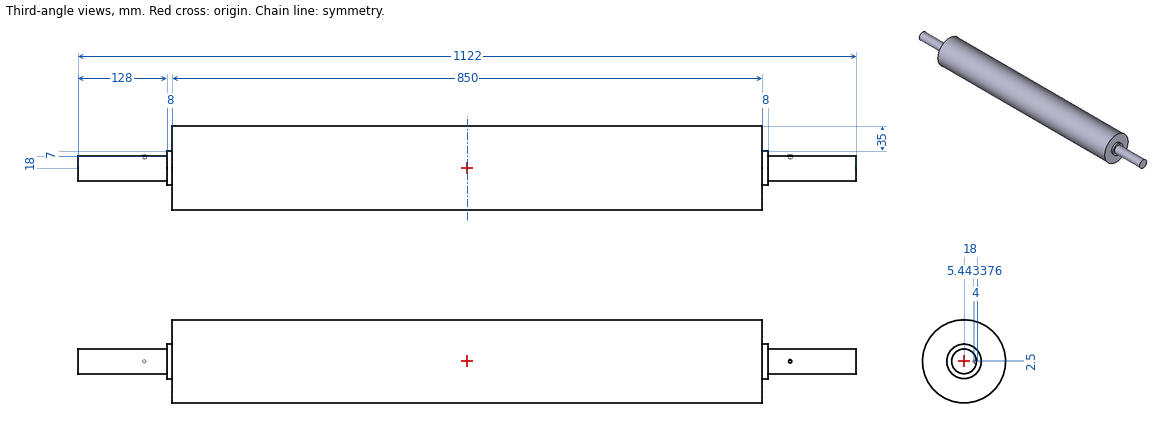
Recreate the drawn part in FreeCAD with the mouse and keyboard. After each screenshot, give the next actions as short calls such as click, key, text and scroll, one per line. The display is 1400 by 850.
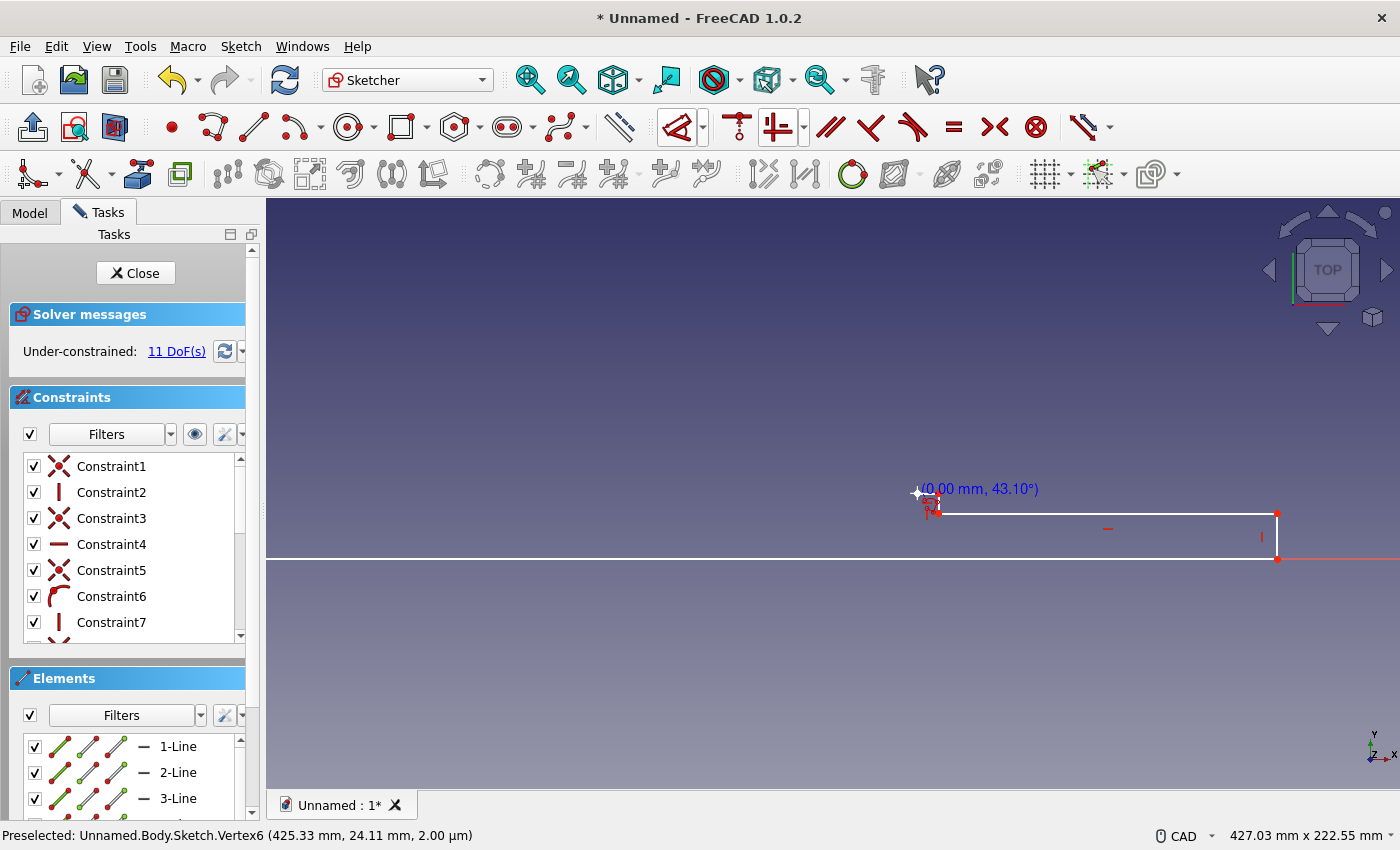
scroll(1011, 497, down, 8)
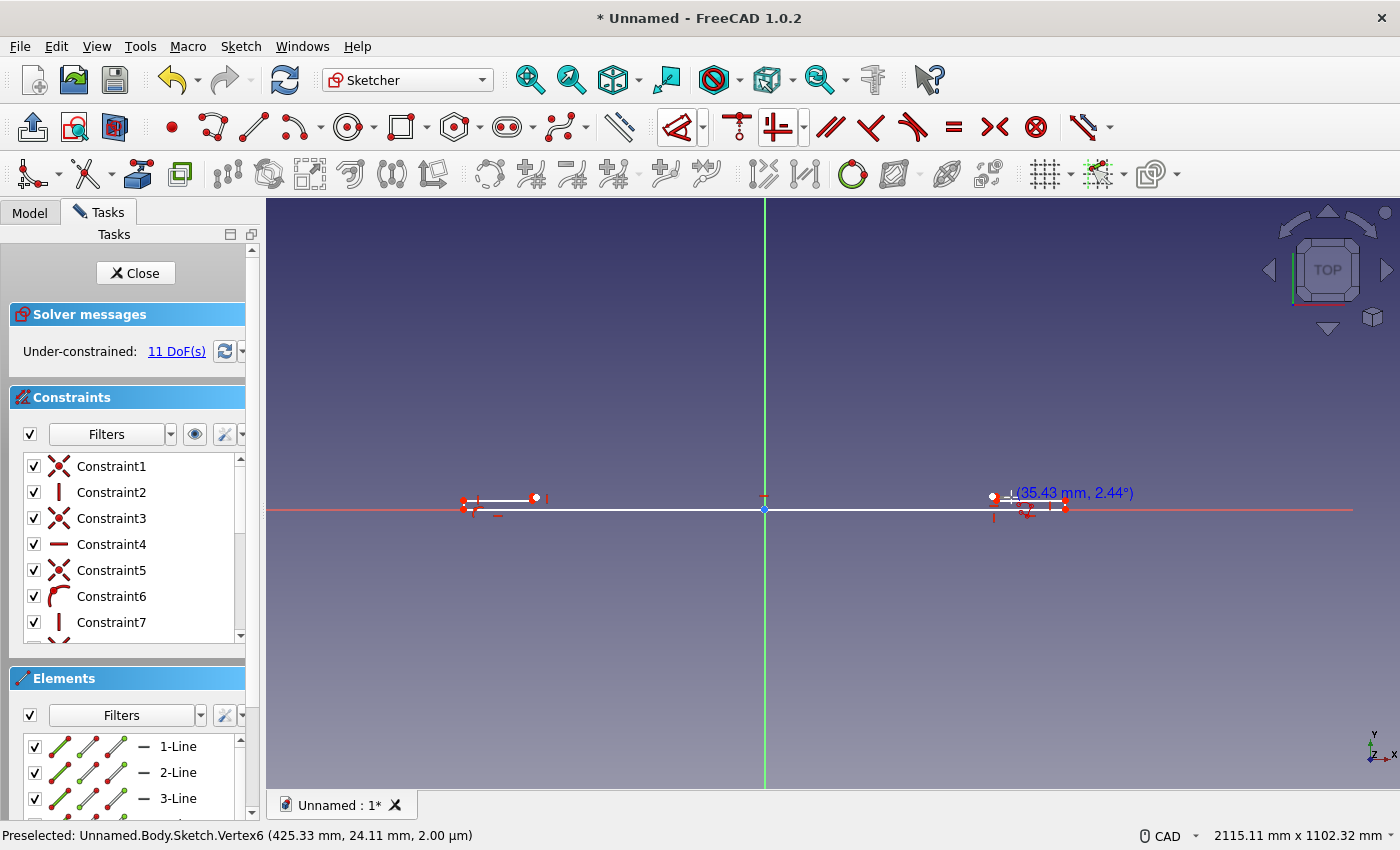
click(993, 478)
click(537, 478)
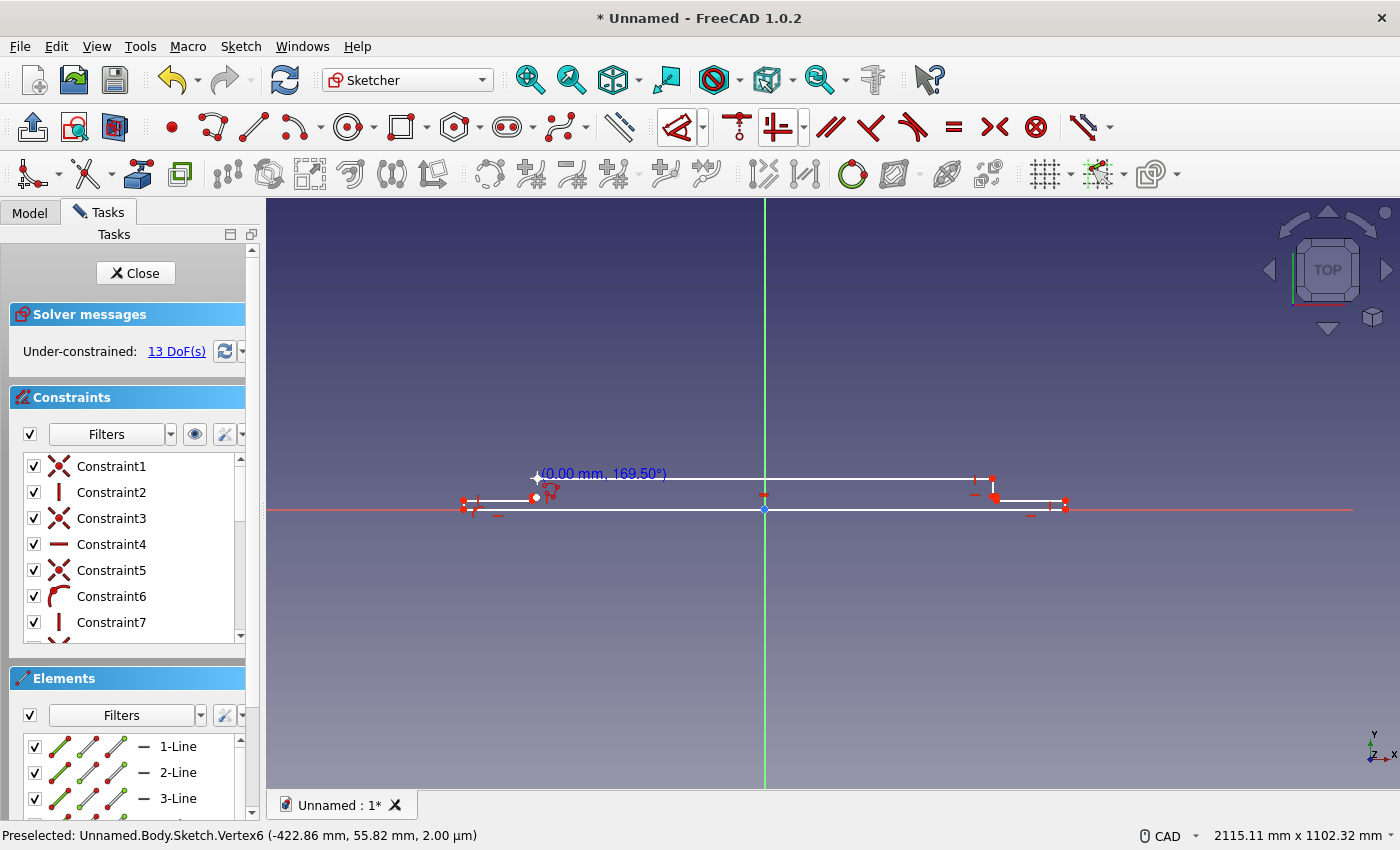
scroll(537, 497, up, 11)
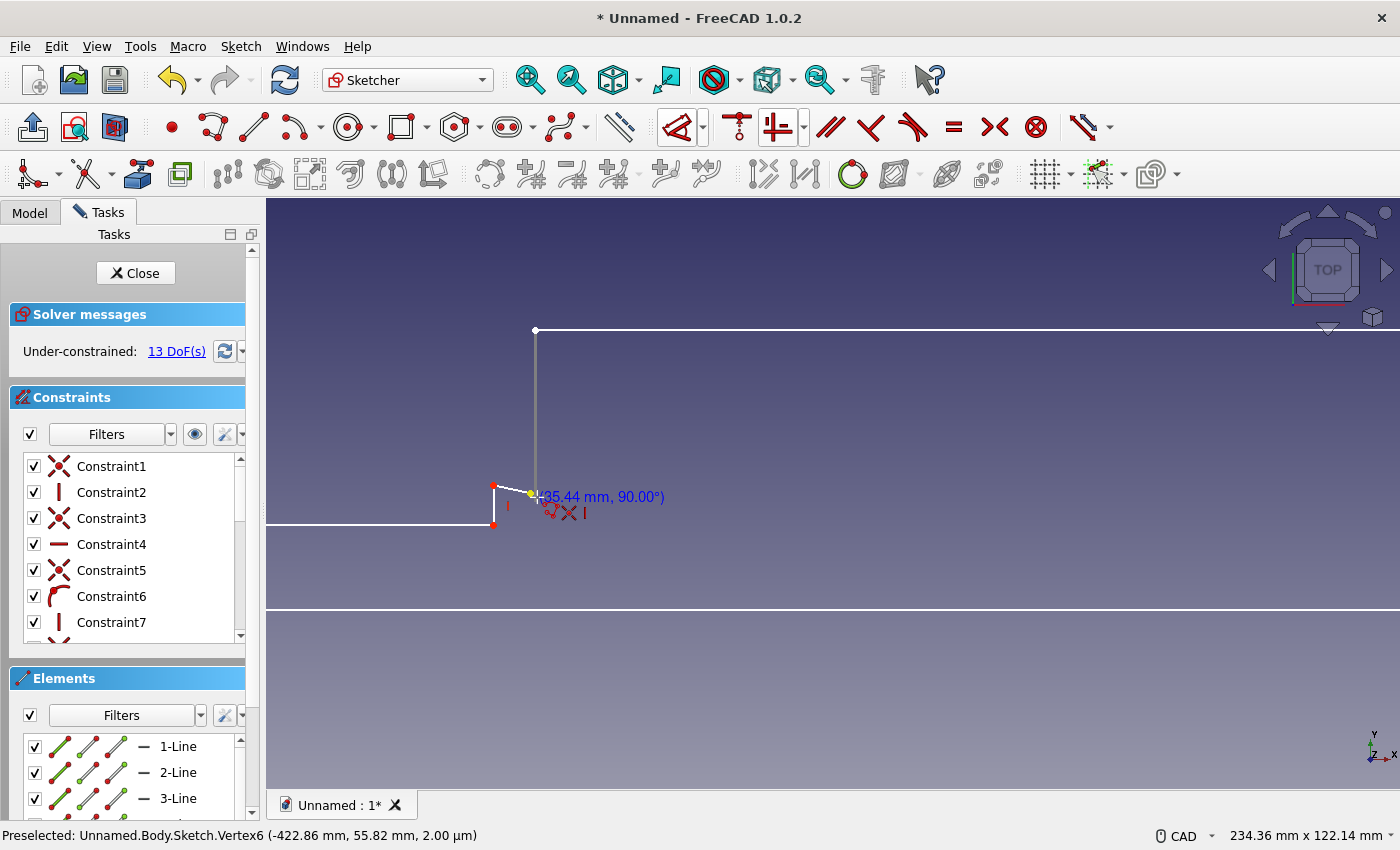
click(531, 484)
key(Escape)
key(Escape)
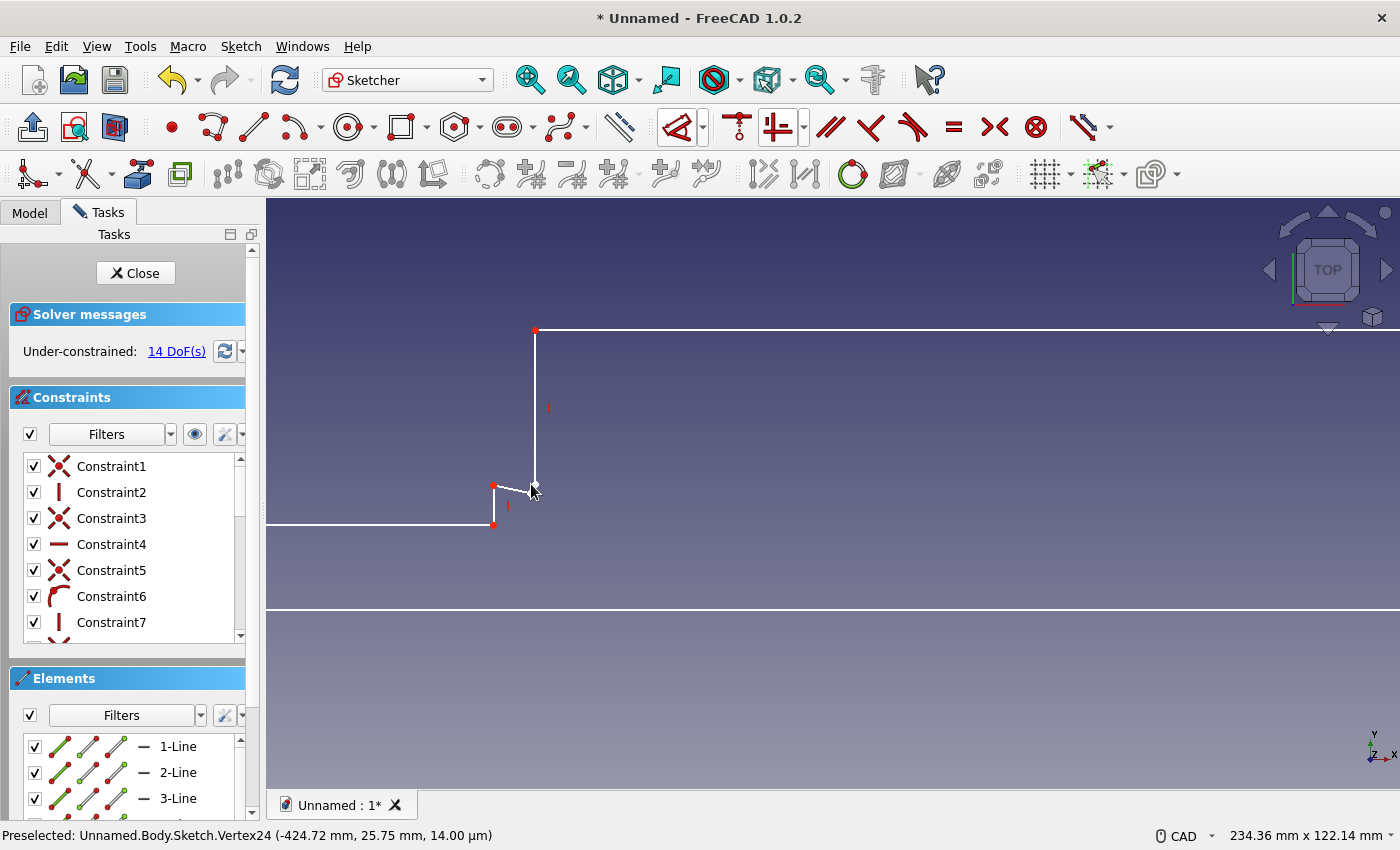
scroll(520, 491, up, 2)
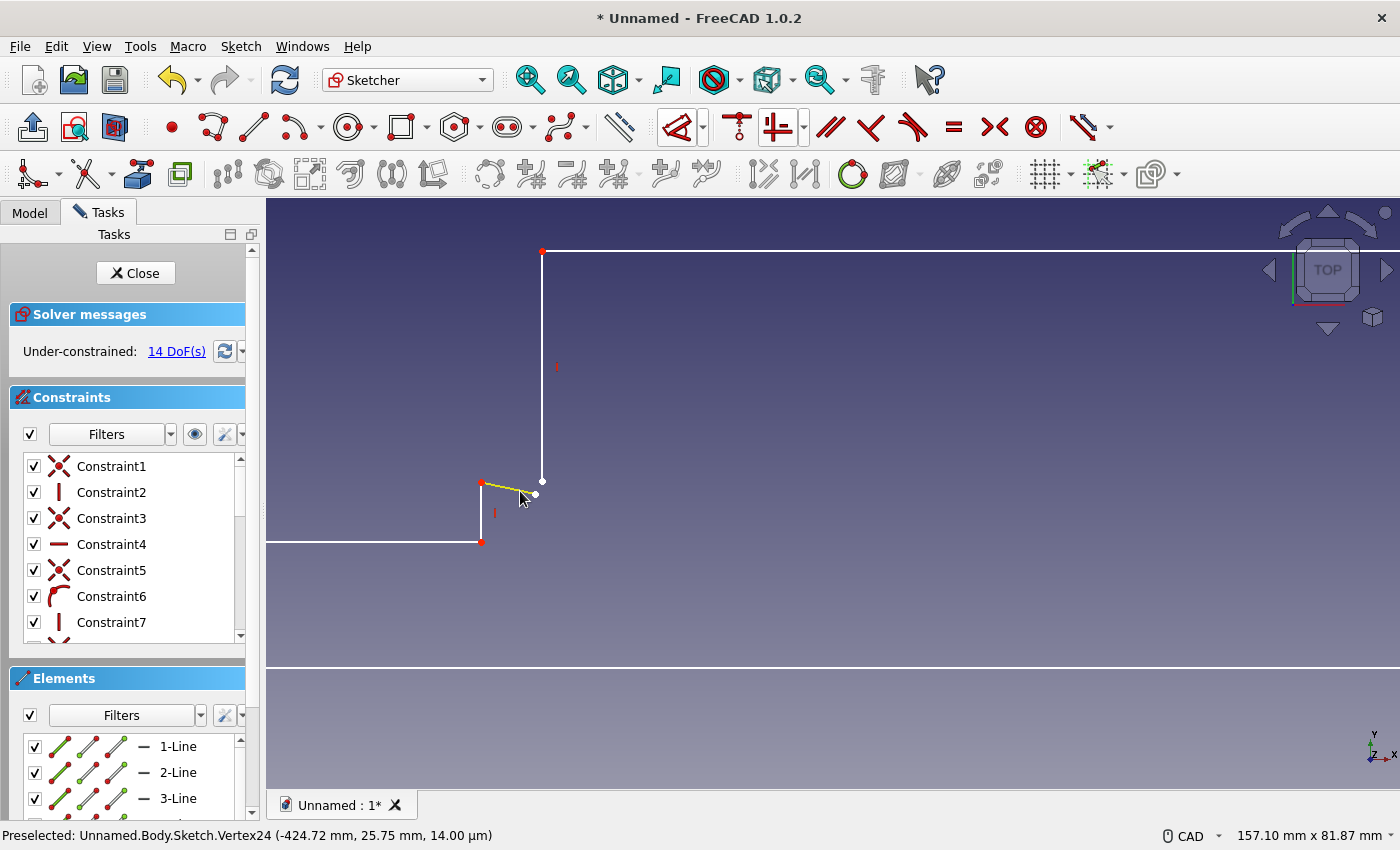
click(519, 491)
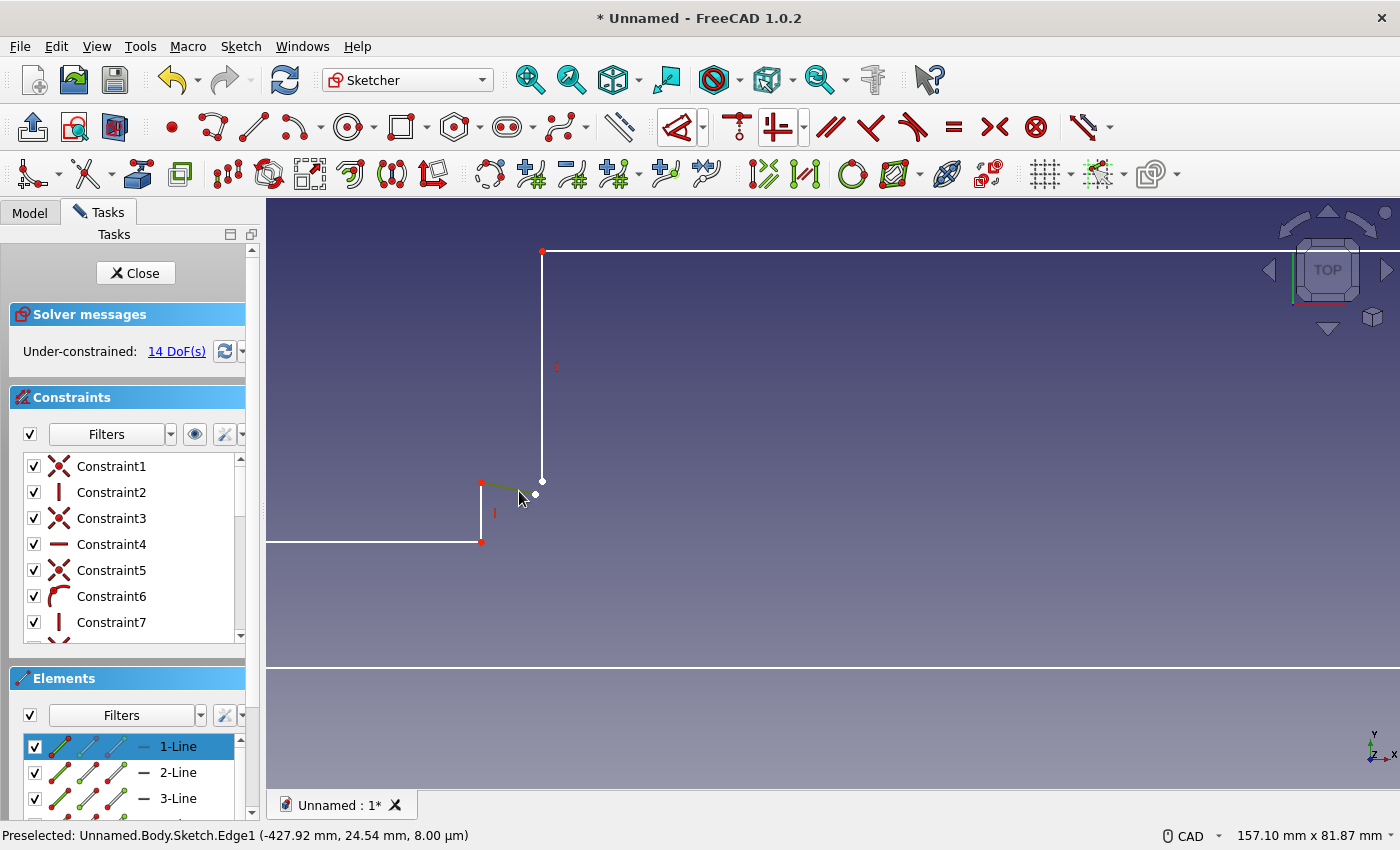
key(h)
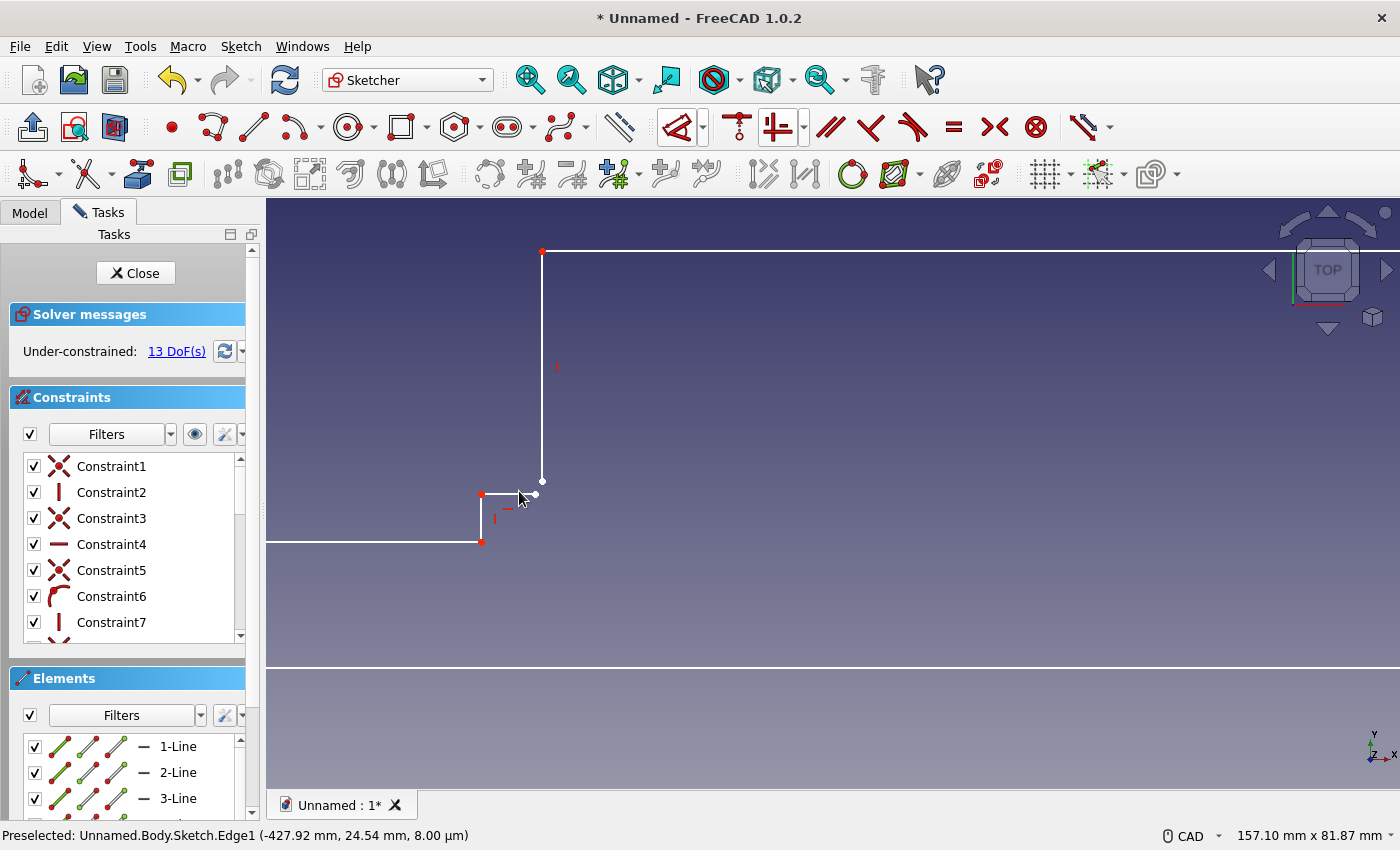
scroll(536, 497, down, 13)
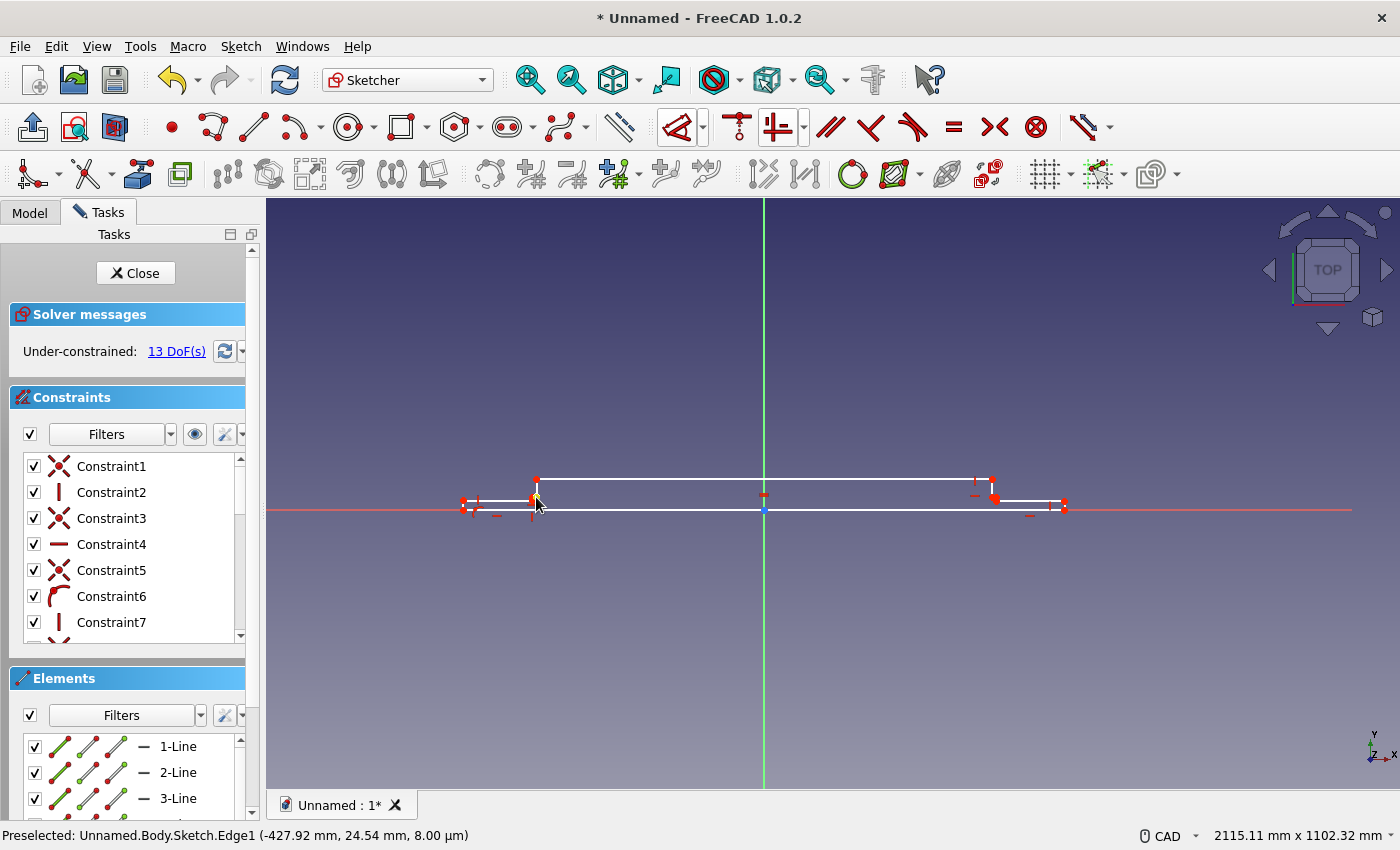
scroll(463, 501, up, 2)